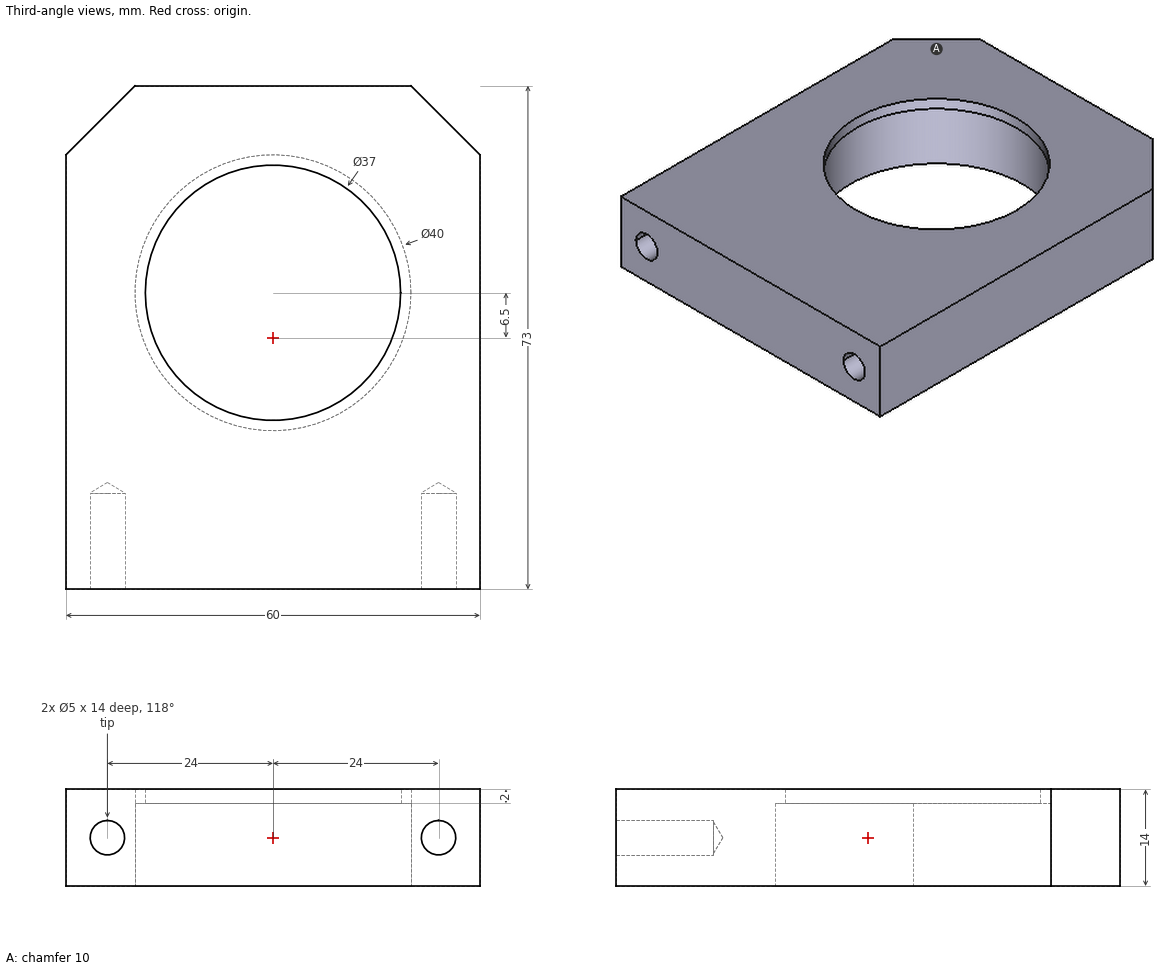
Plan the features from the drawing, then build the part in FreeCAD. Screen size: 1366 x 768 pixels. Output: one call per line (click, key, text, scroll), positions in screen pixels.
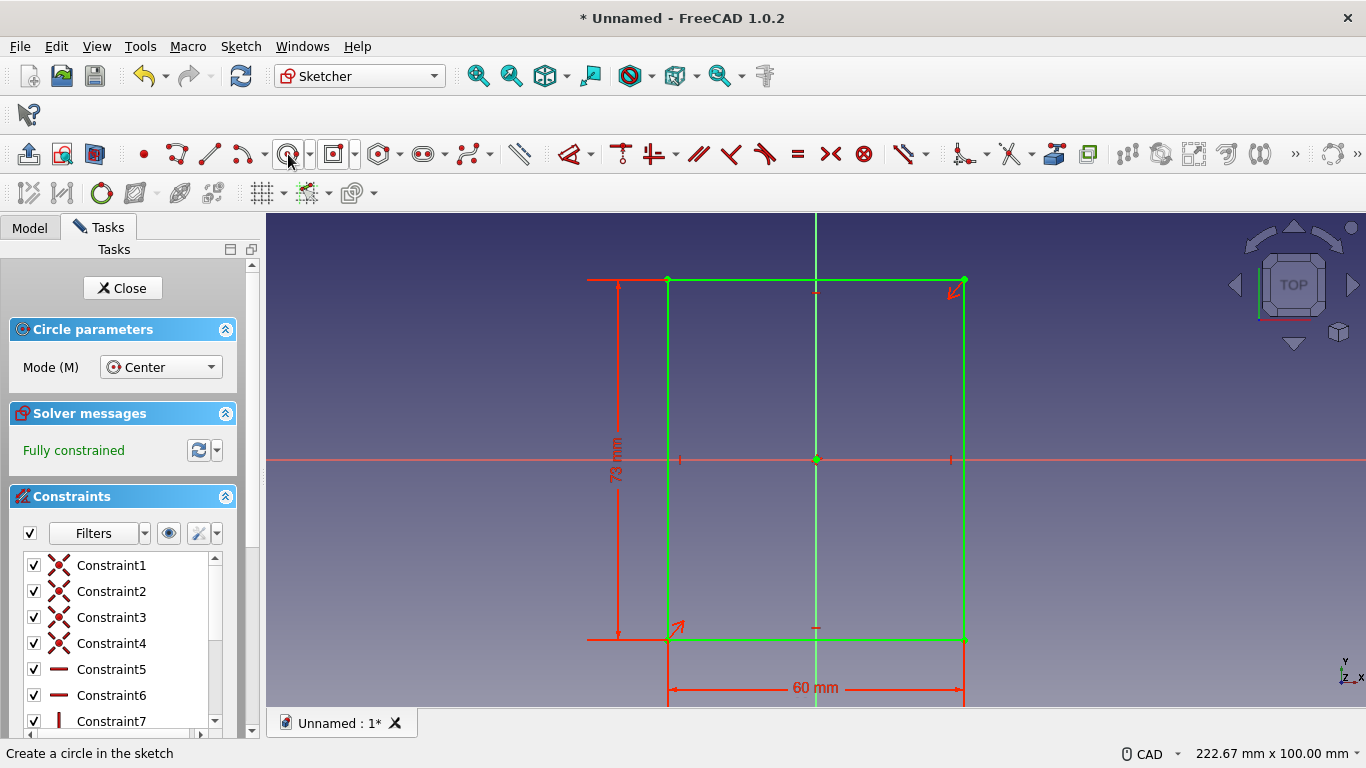
click(816, 428)
move(886, 358)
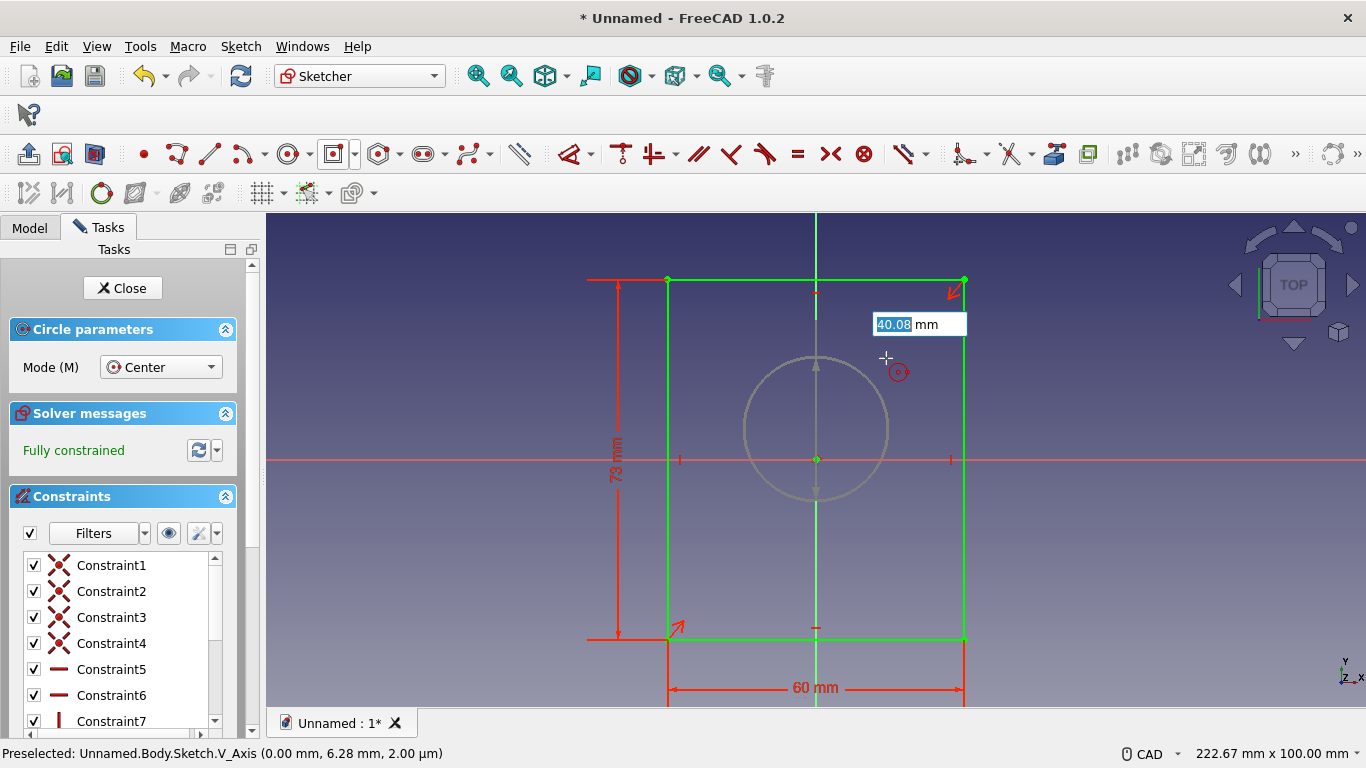
text(40)
key(Return)
key(Escape)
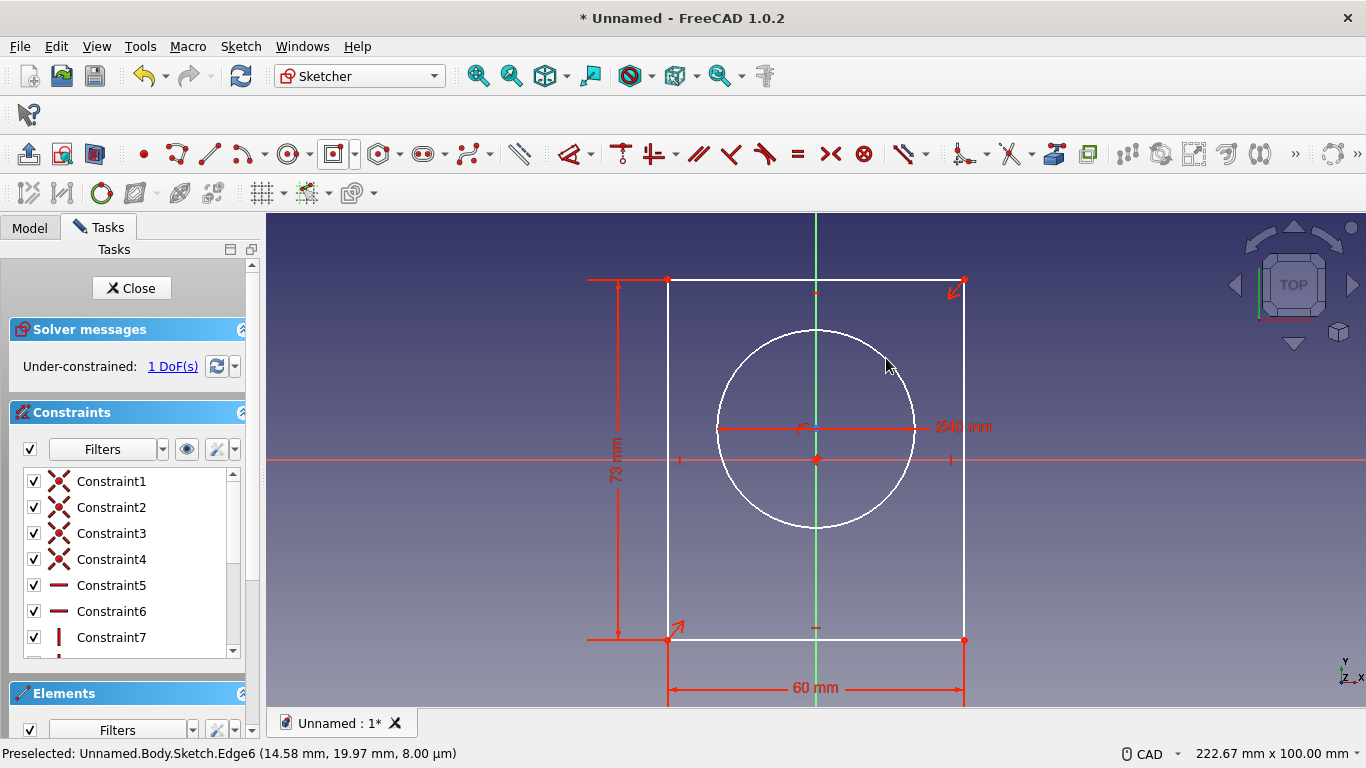
click(568, 154)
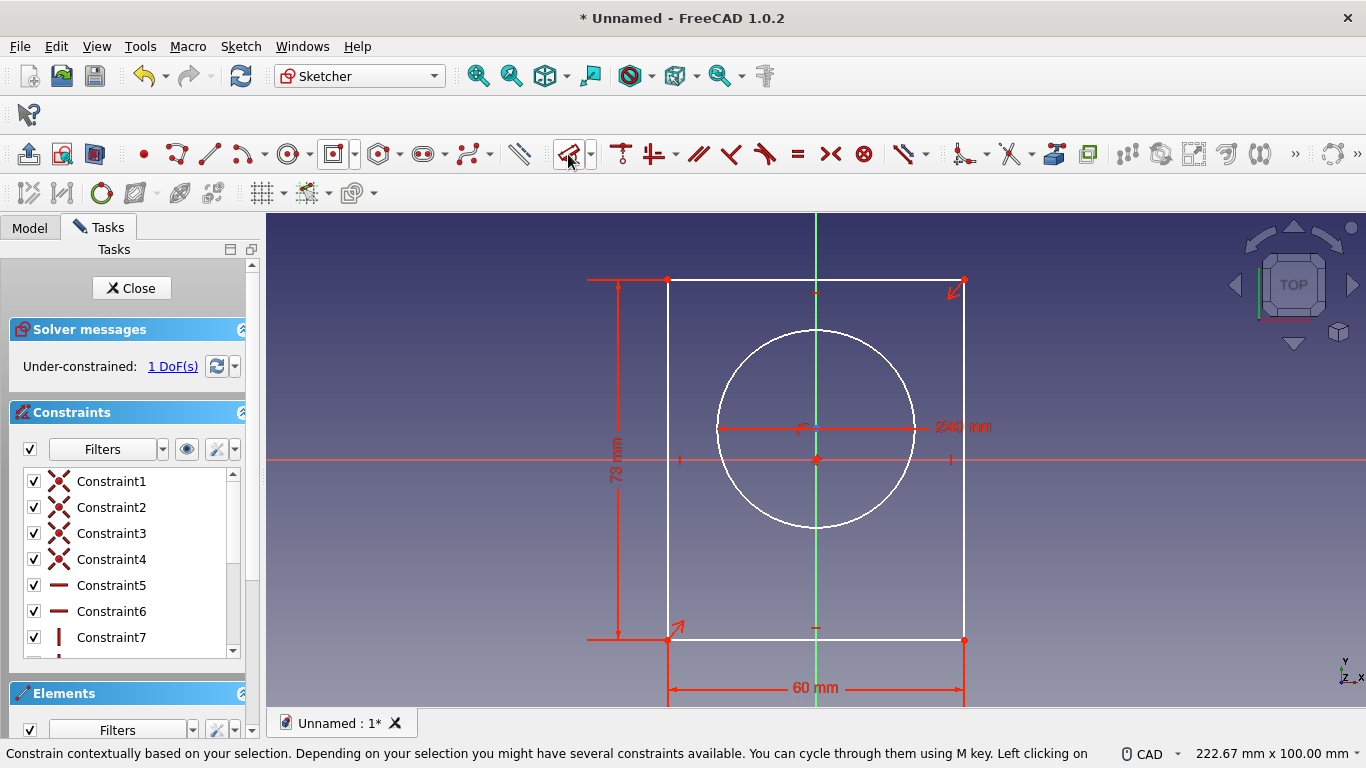
scroll(816, 429, up, 2)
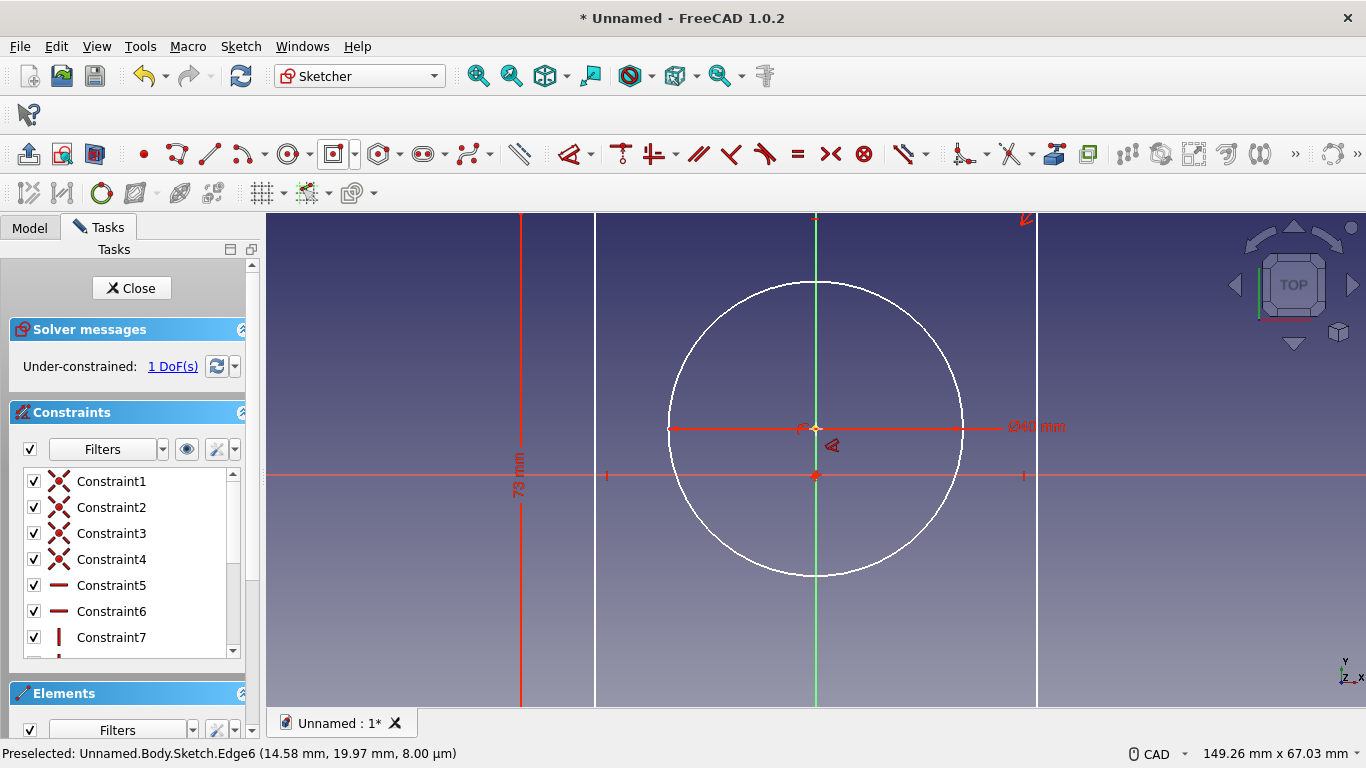
click(816, 429)
click(850, 452)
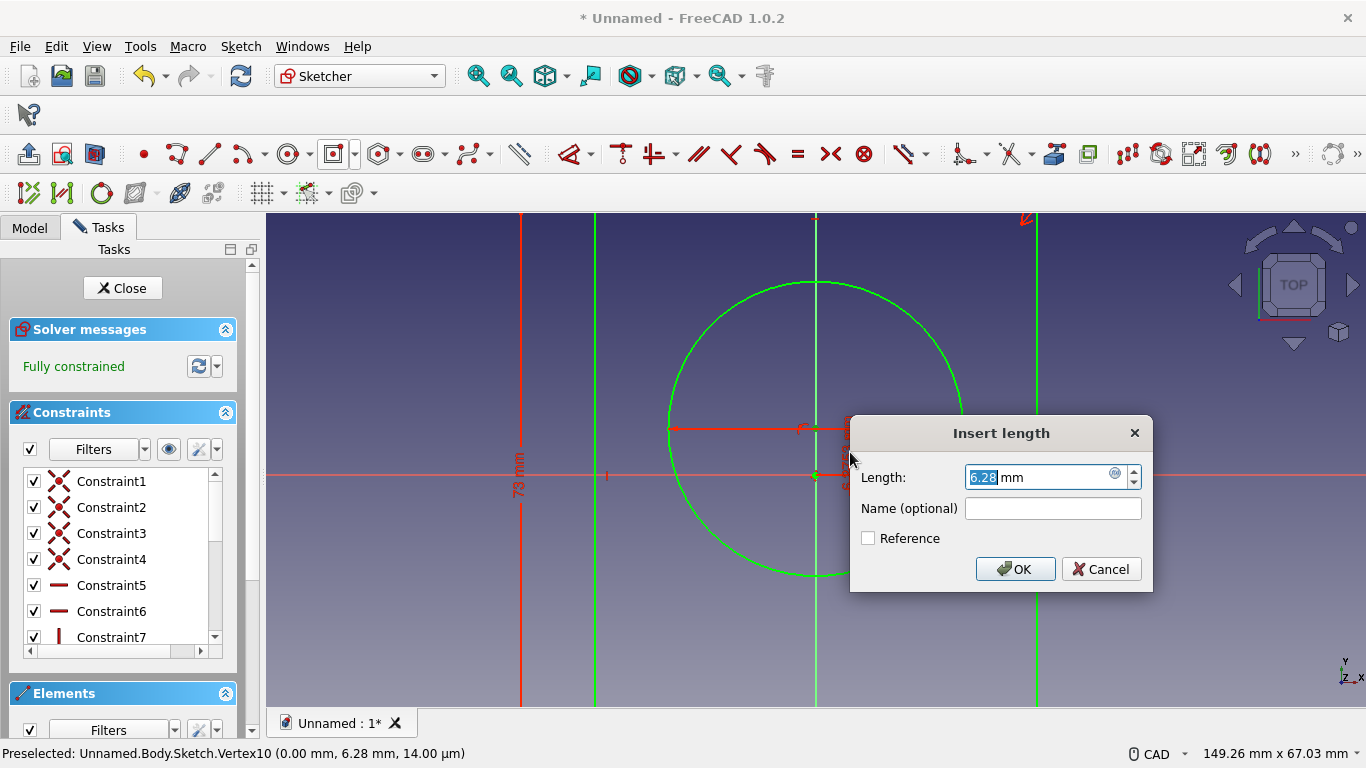
text(6.5)
key(Return)
key(Escape)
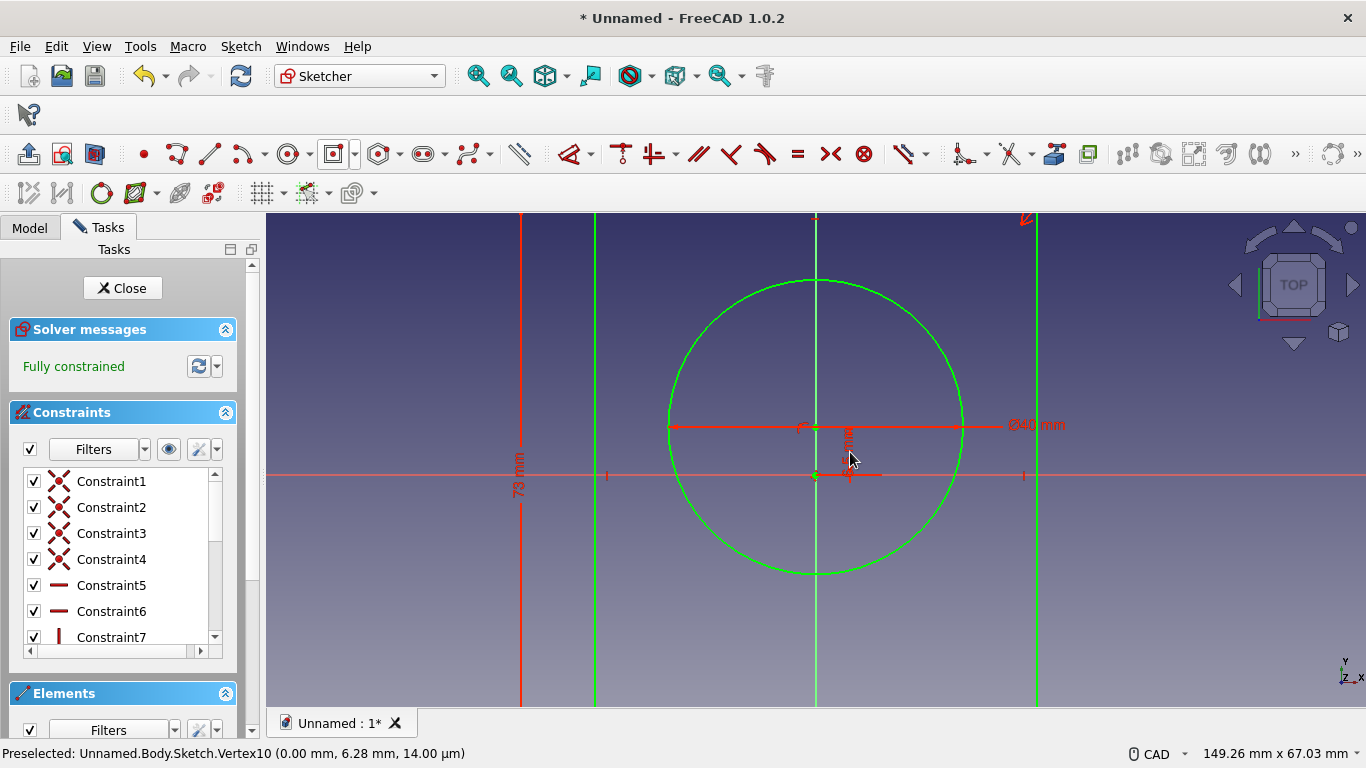
click(123, 288)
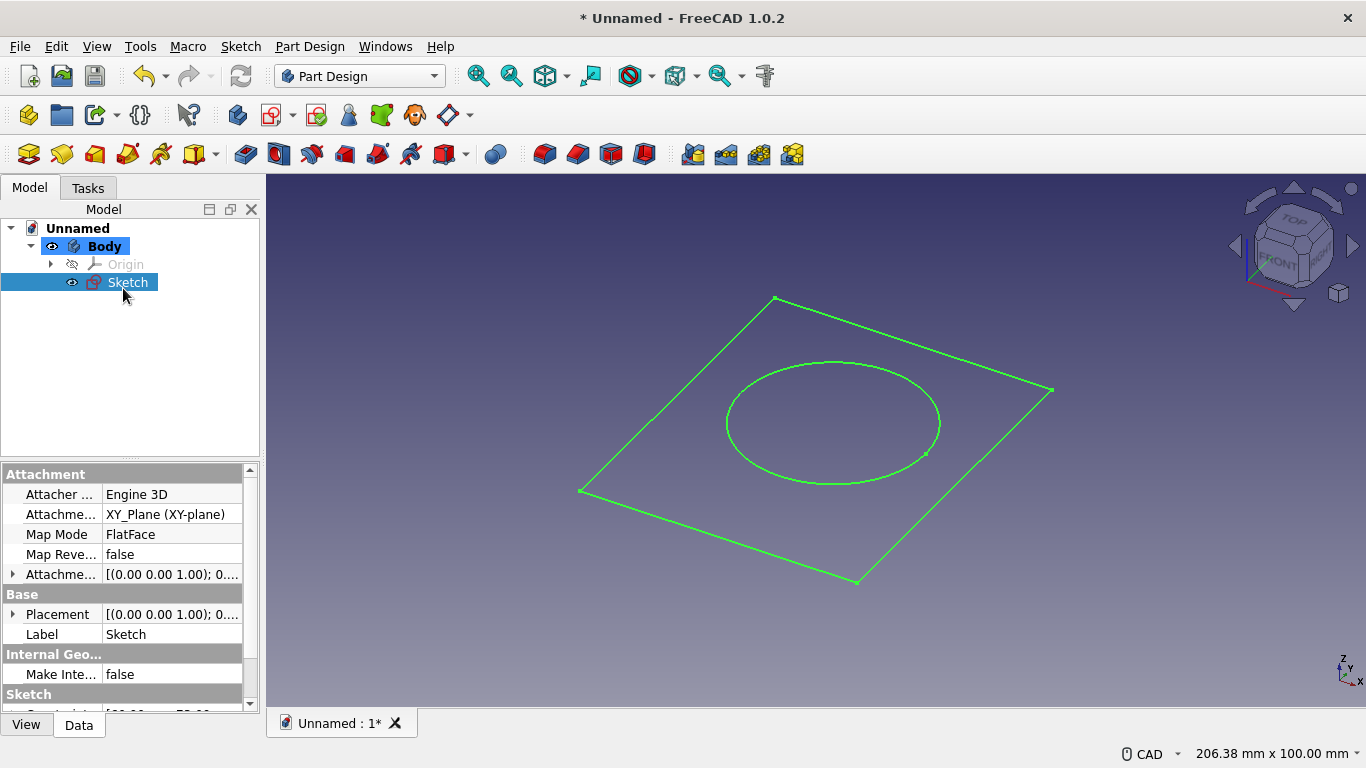
click(29, 154)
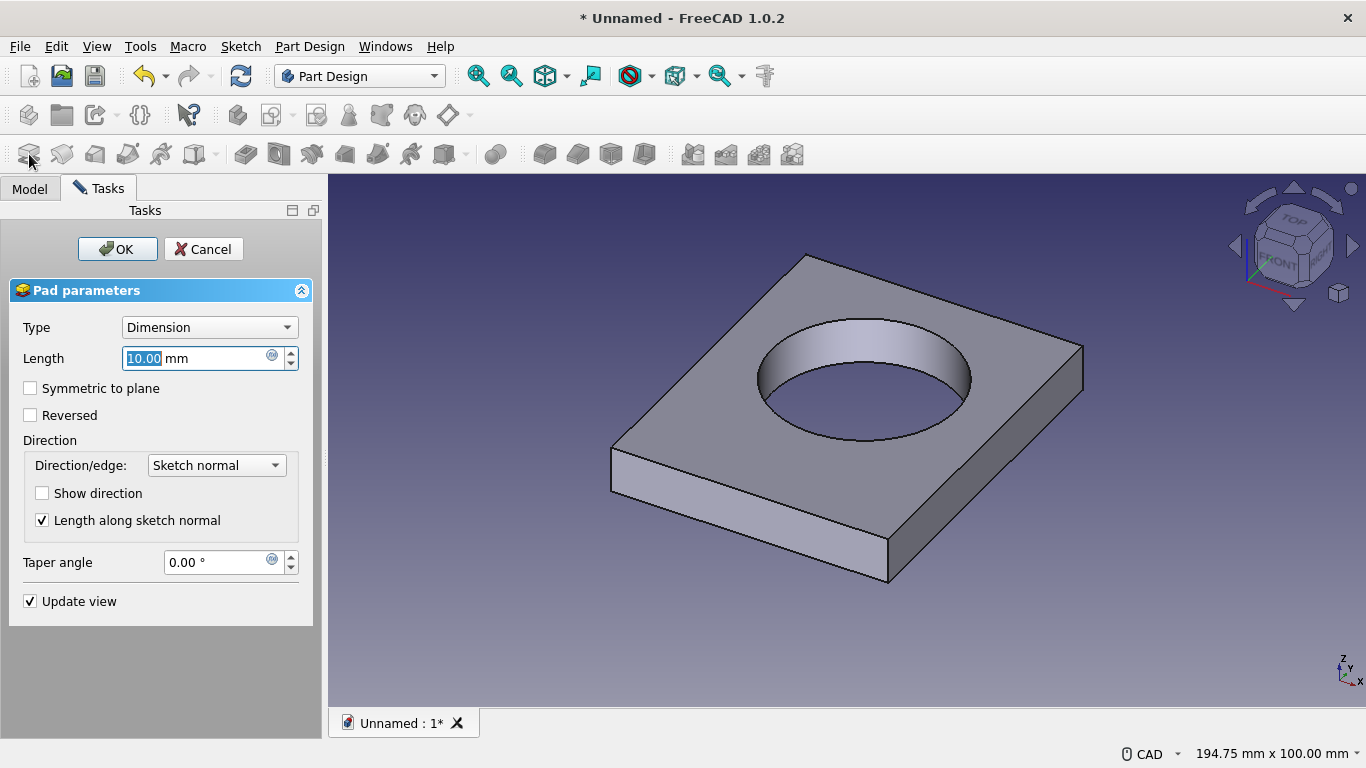
text(14)
key(Tab)